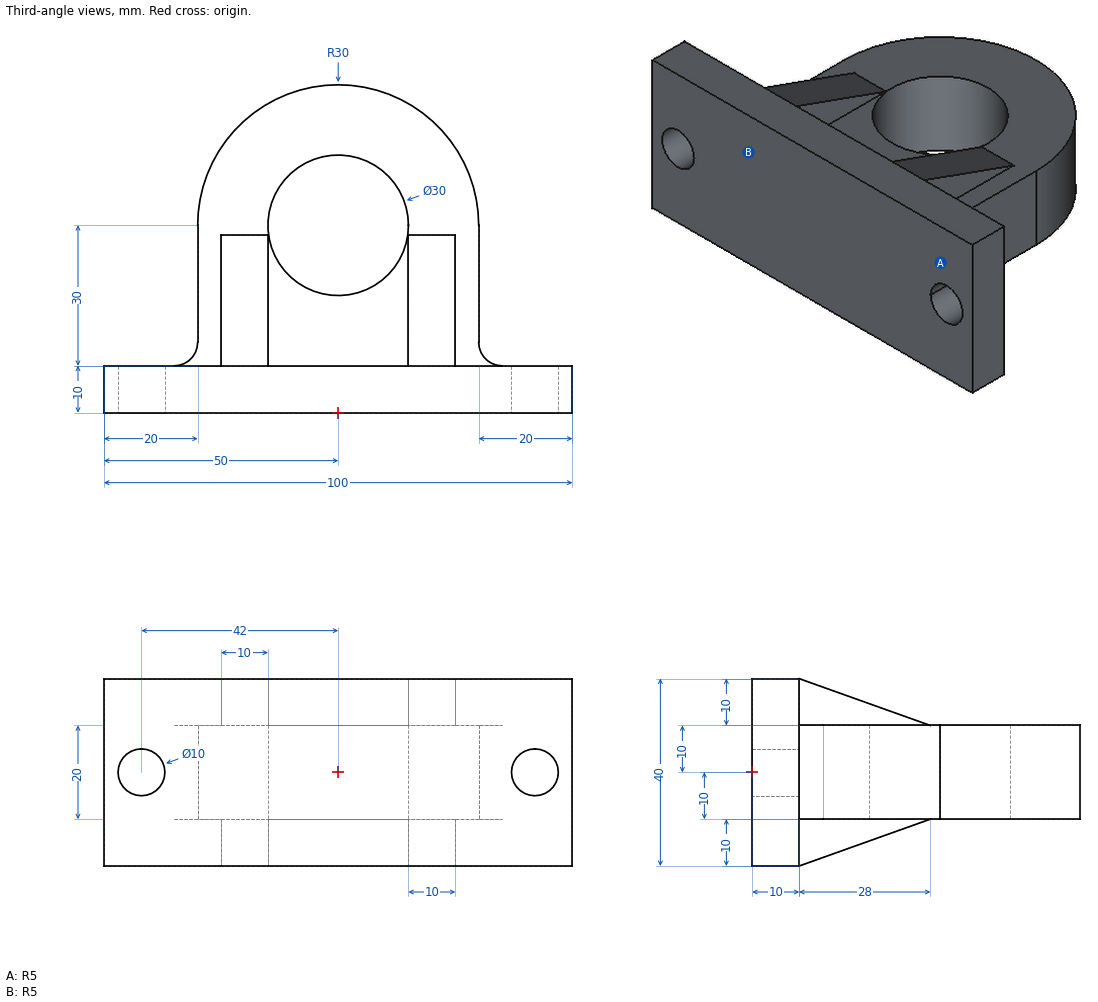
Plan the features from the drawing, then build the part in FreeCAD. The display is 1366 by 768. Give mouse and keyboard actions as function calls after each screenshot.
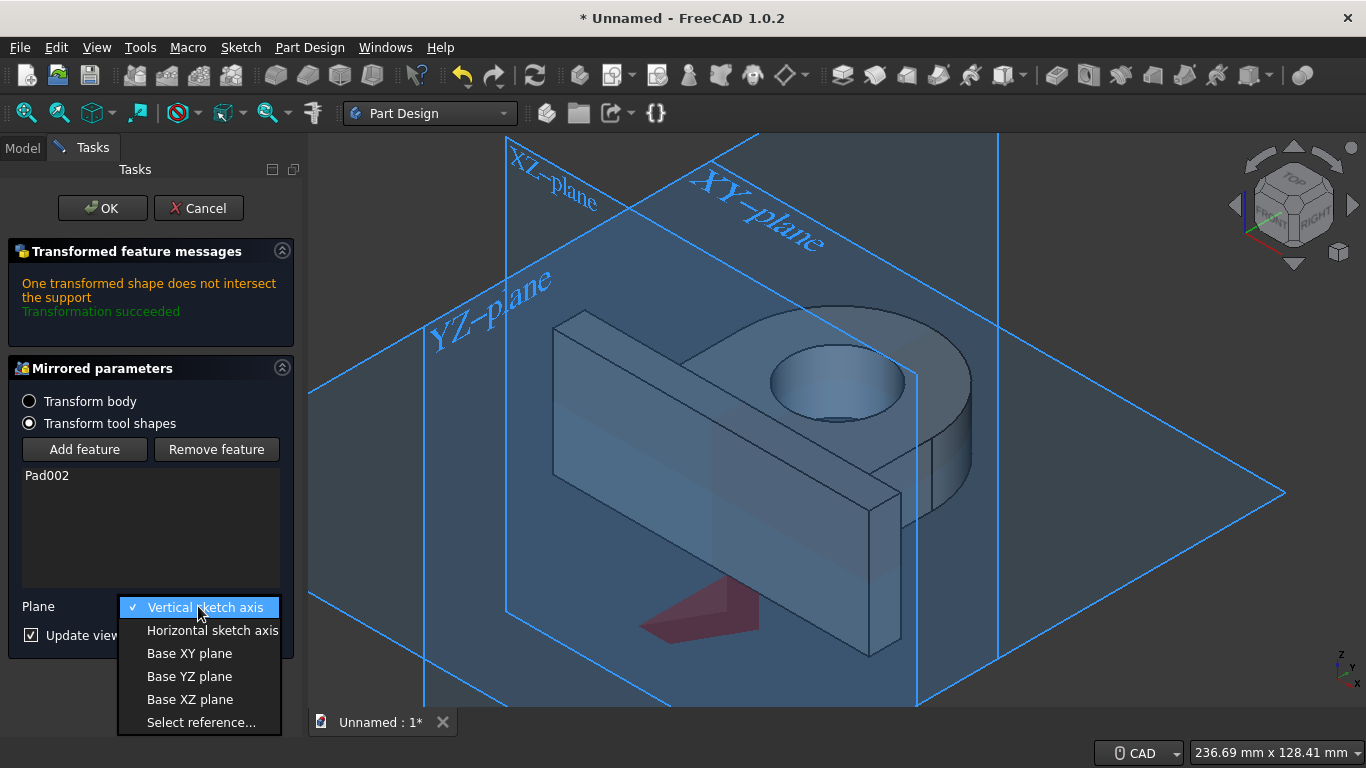
click(198, 654)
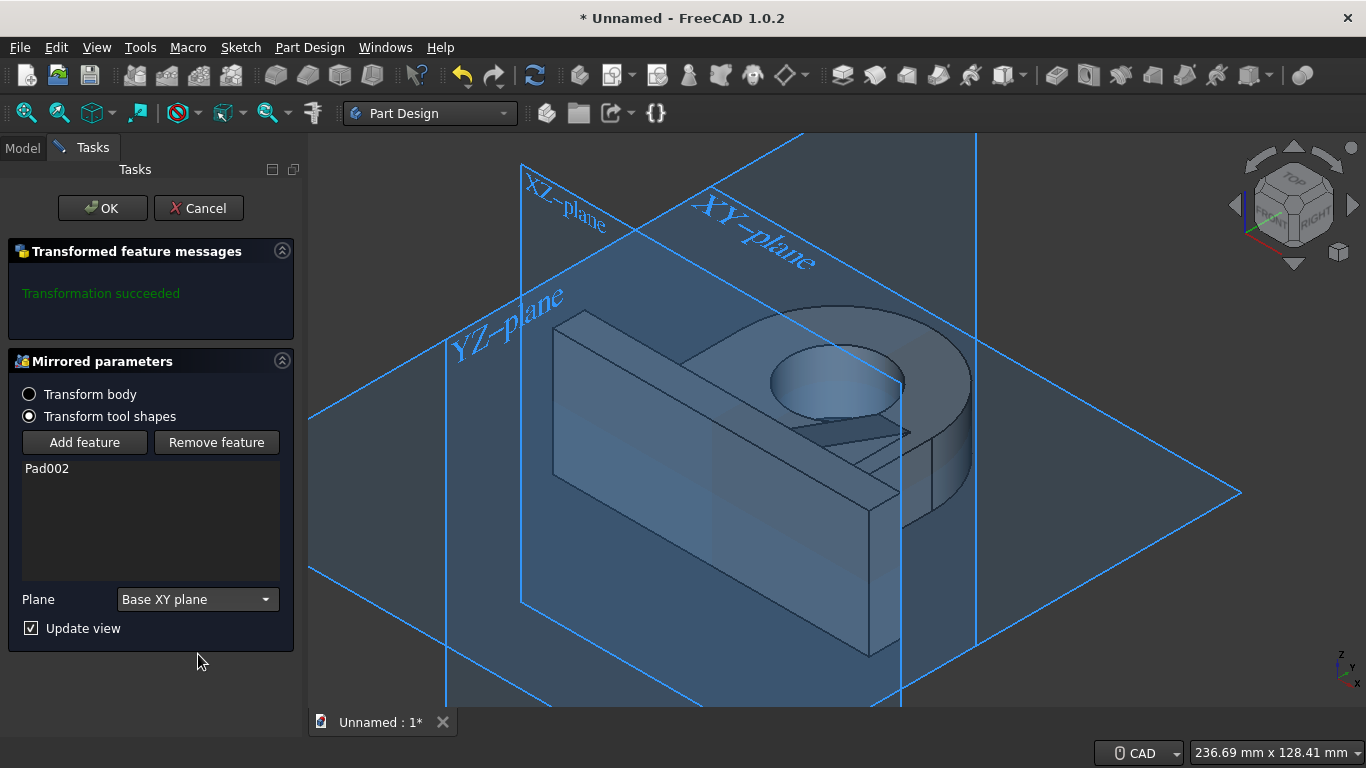
click(103, 208)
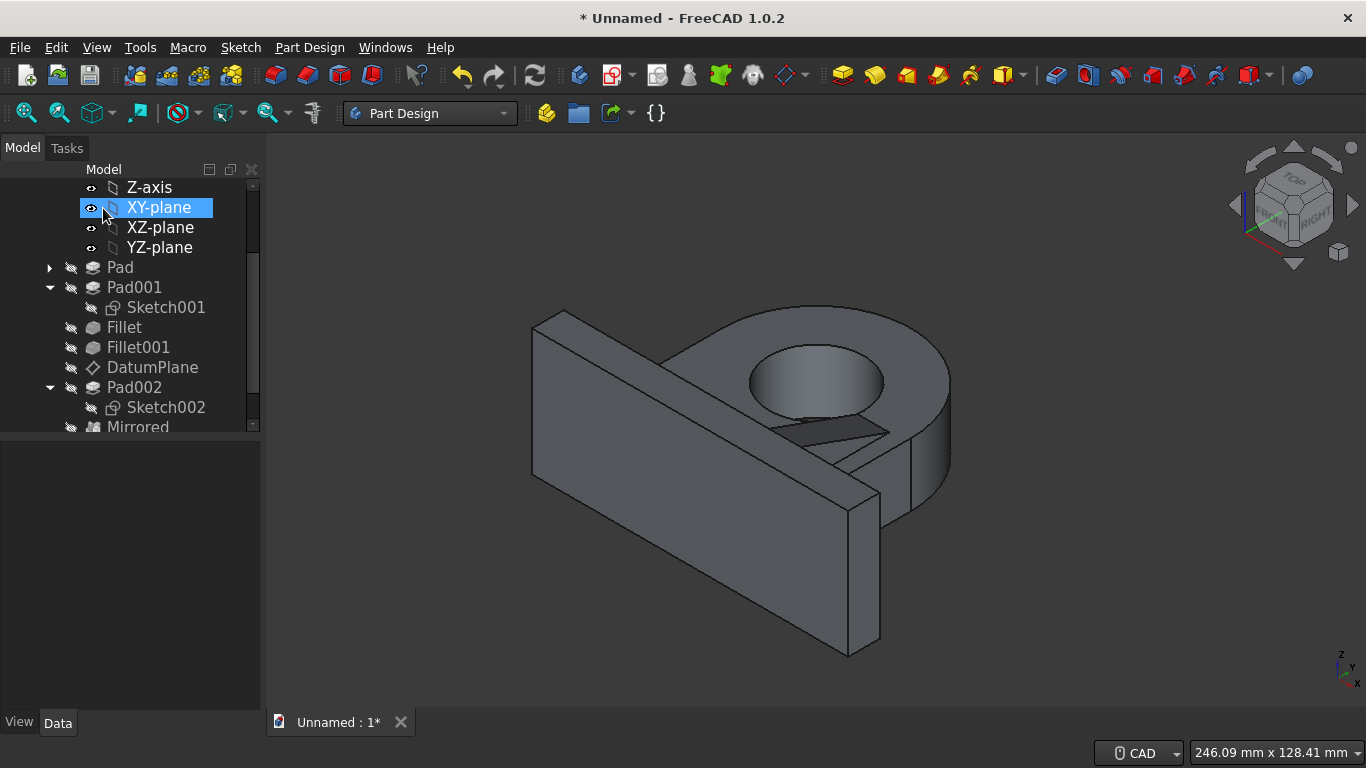
key(6)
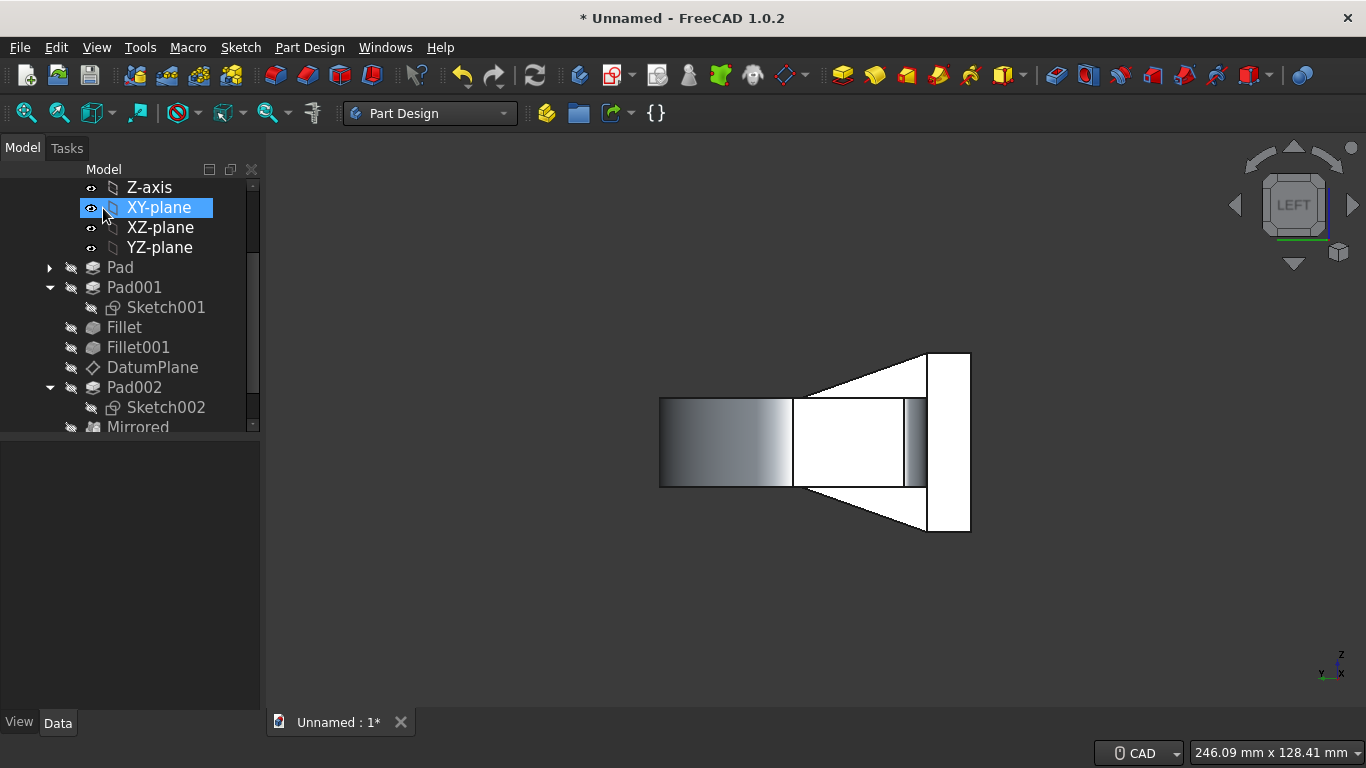
click(28, 114)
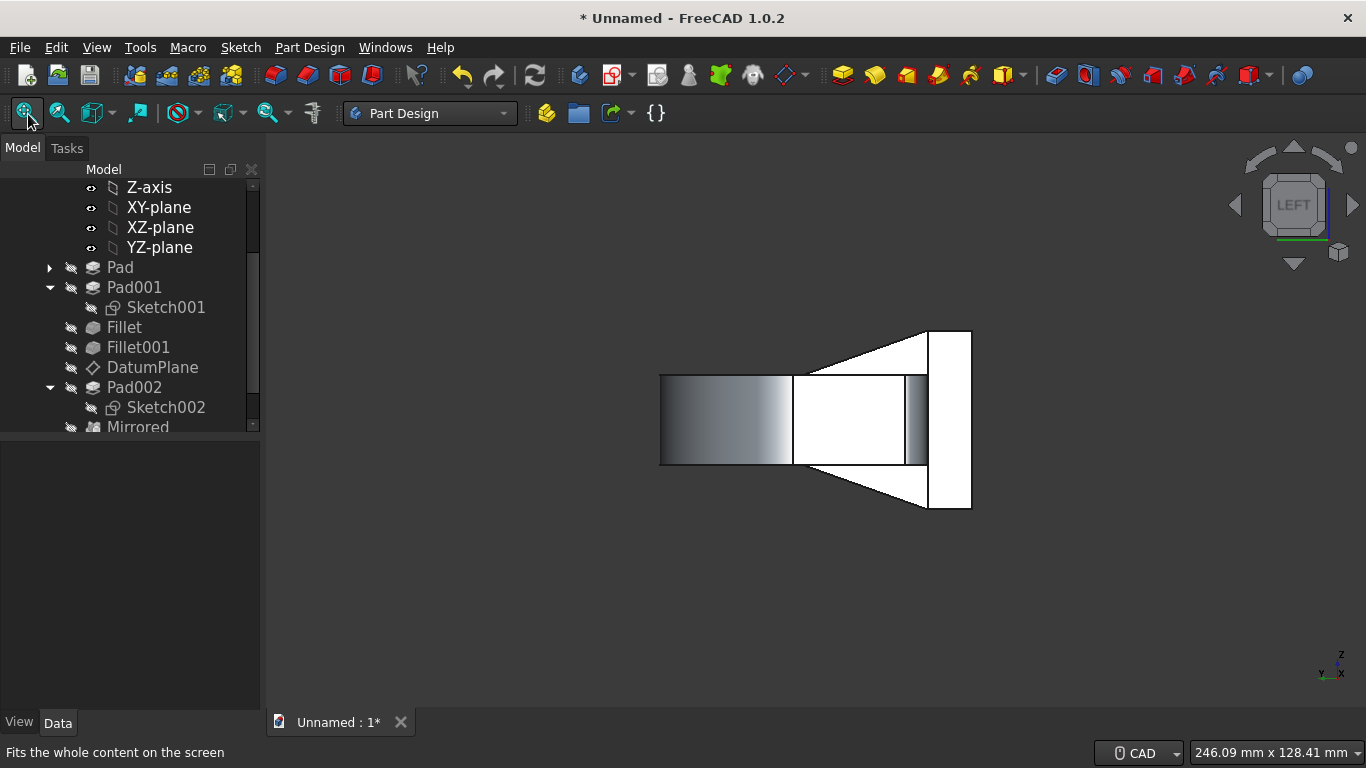
click(901, 480)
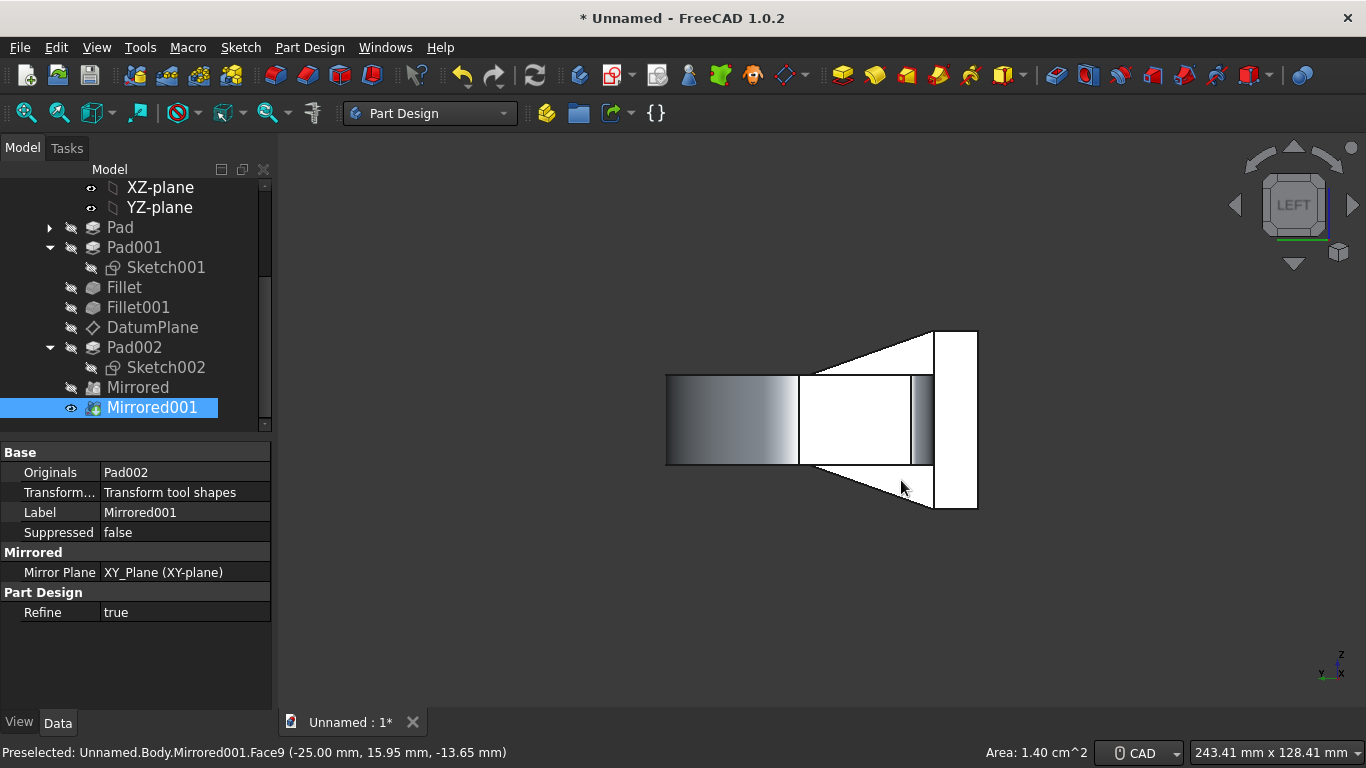
click(612, 76)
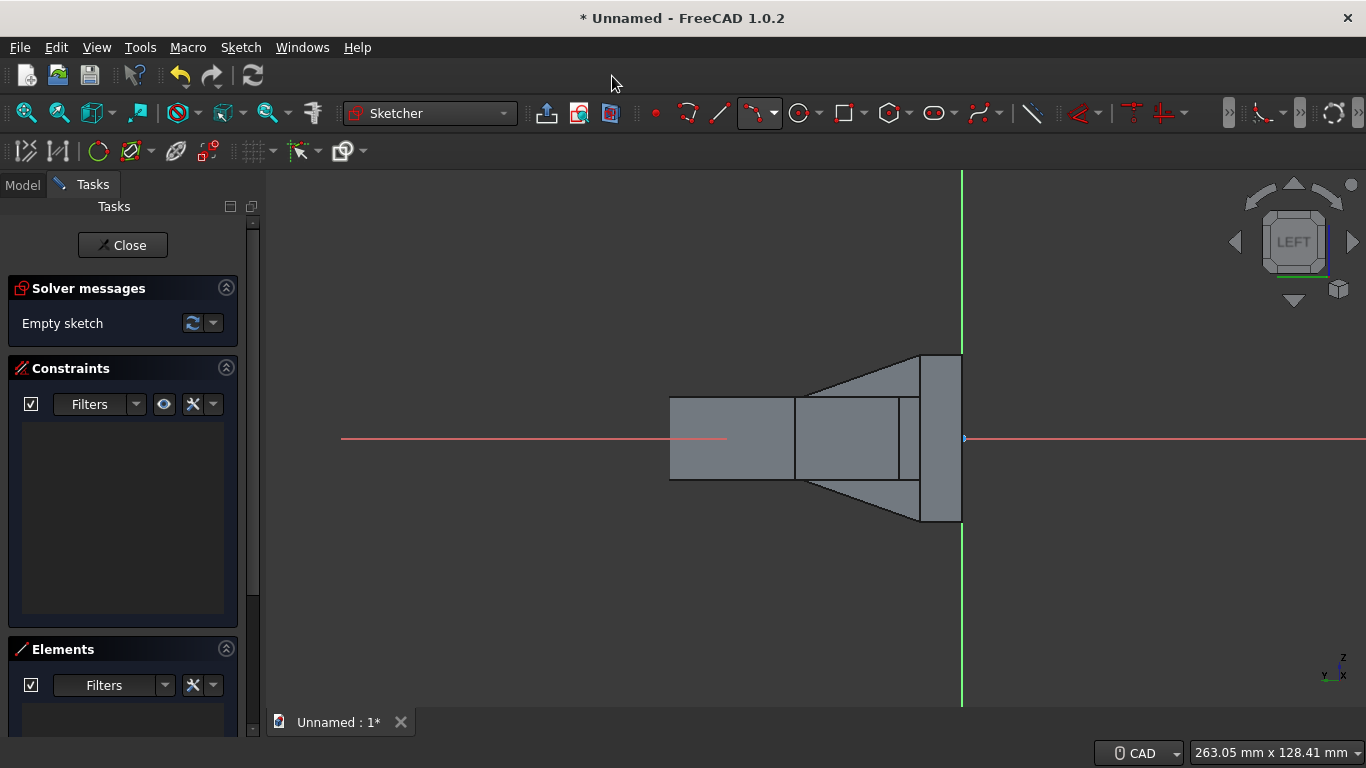
scroll(927, 383, up, 7)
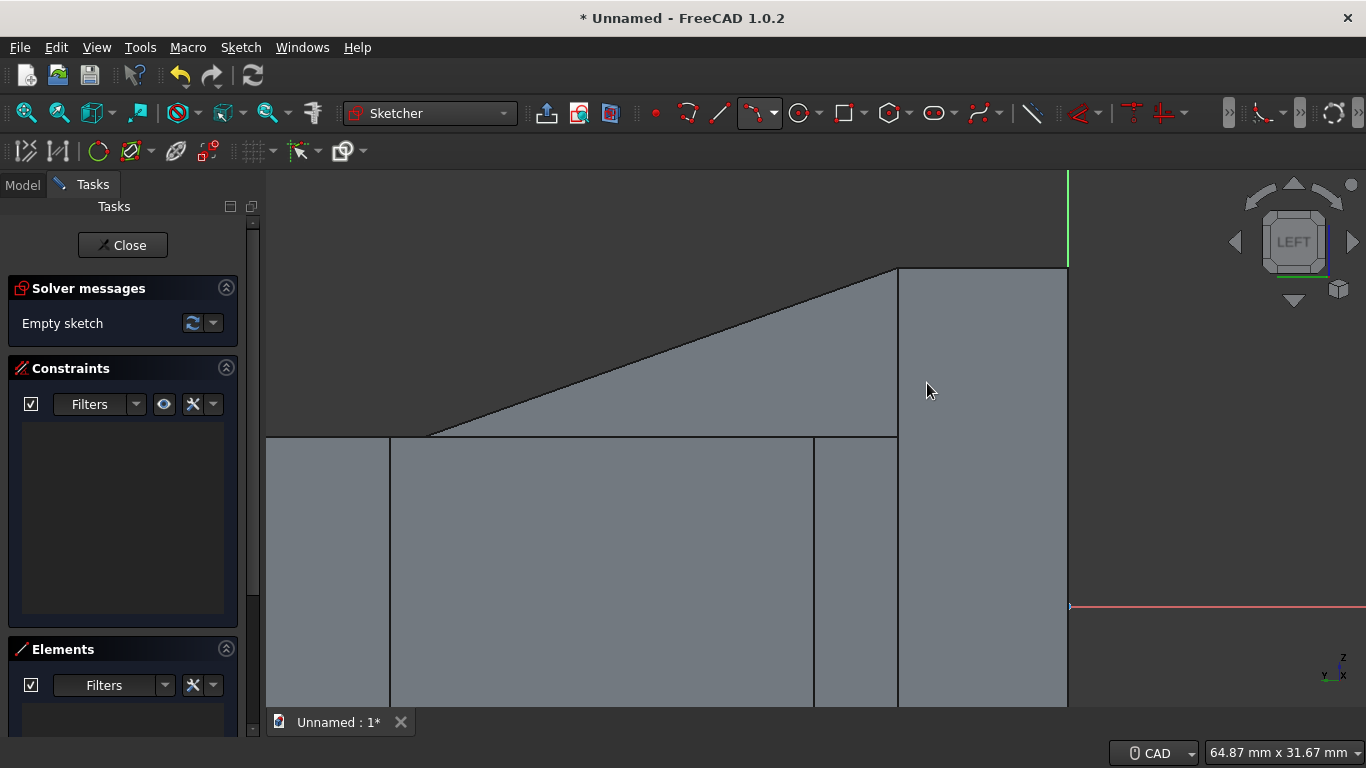
click(688, 114)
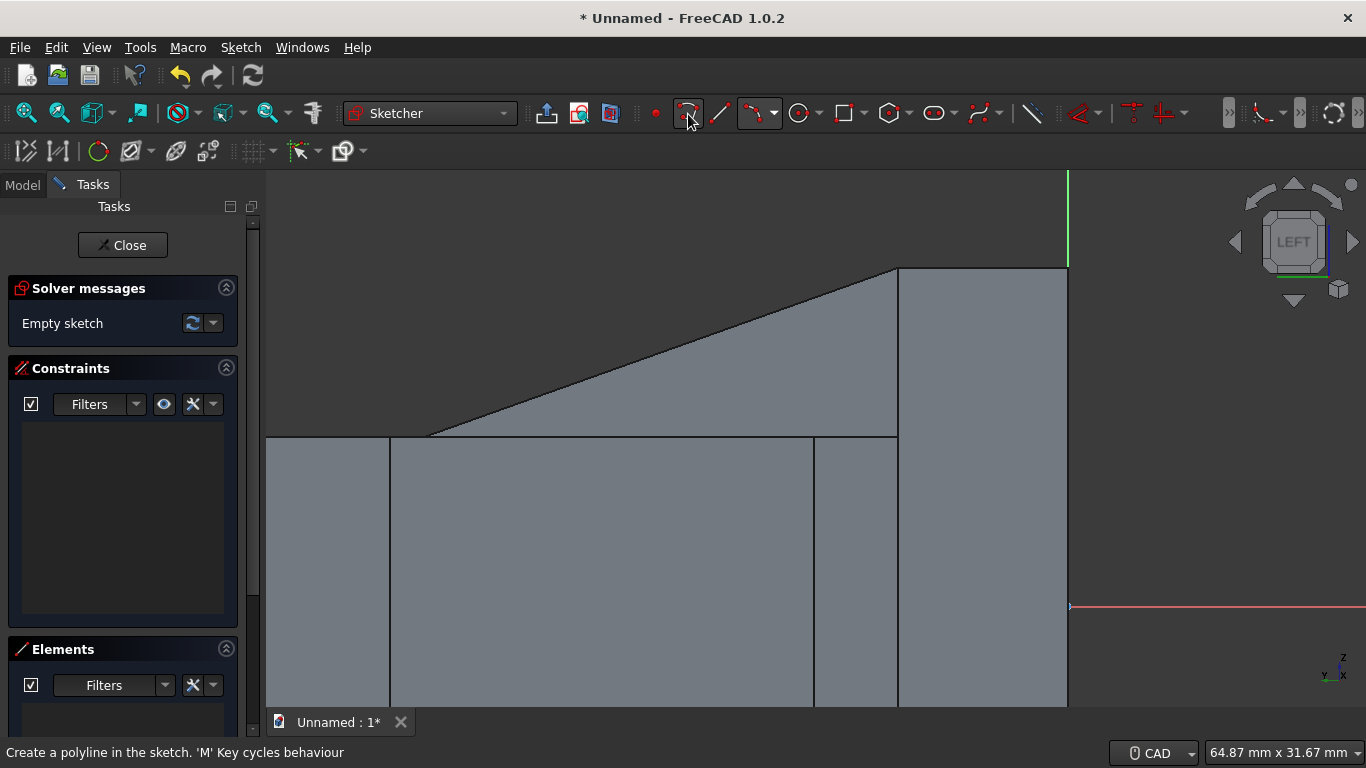
click(898, 437)
click(898, 268)
click(424, 437)
click(898, 438)
key(Escape)
key(Escape)